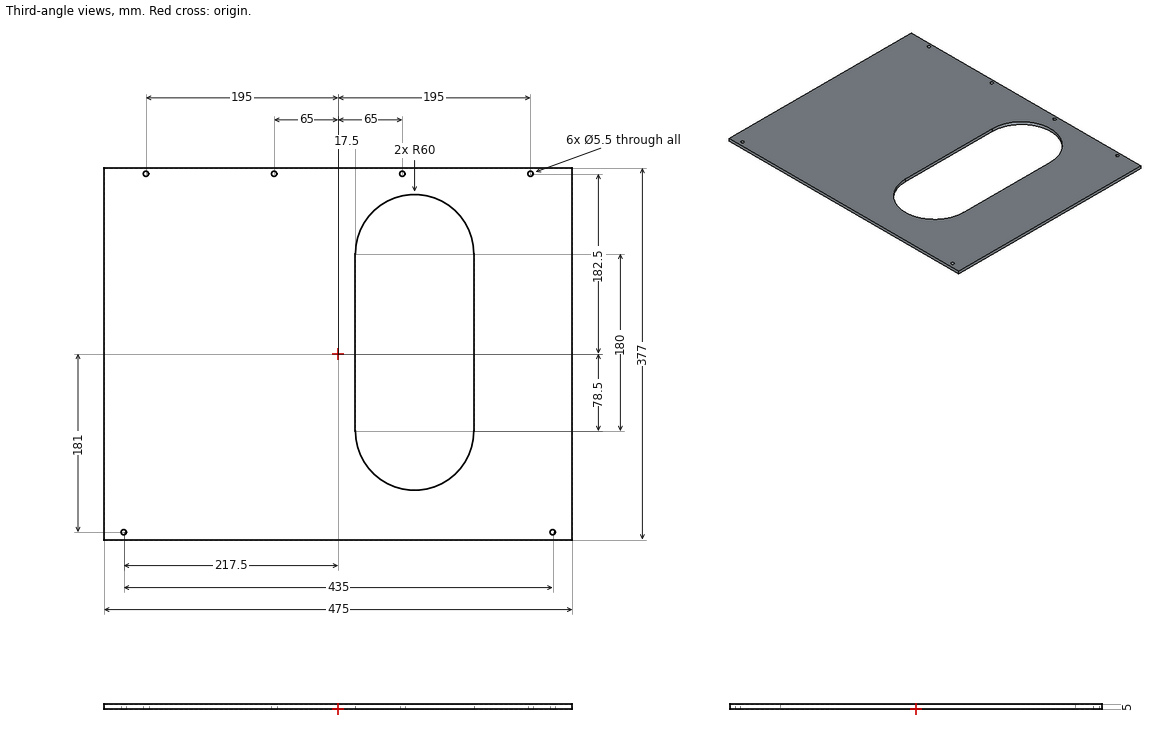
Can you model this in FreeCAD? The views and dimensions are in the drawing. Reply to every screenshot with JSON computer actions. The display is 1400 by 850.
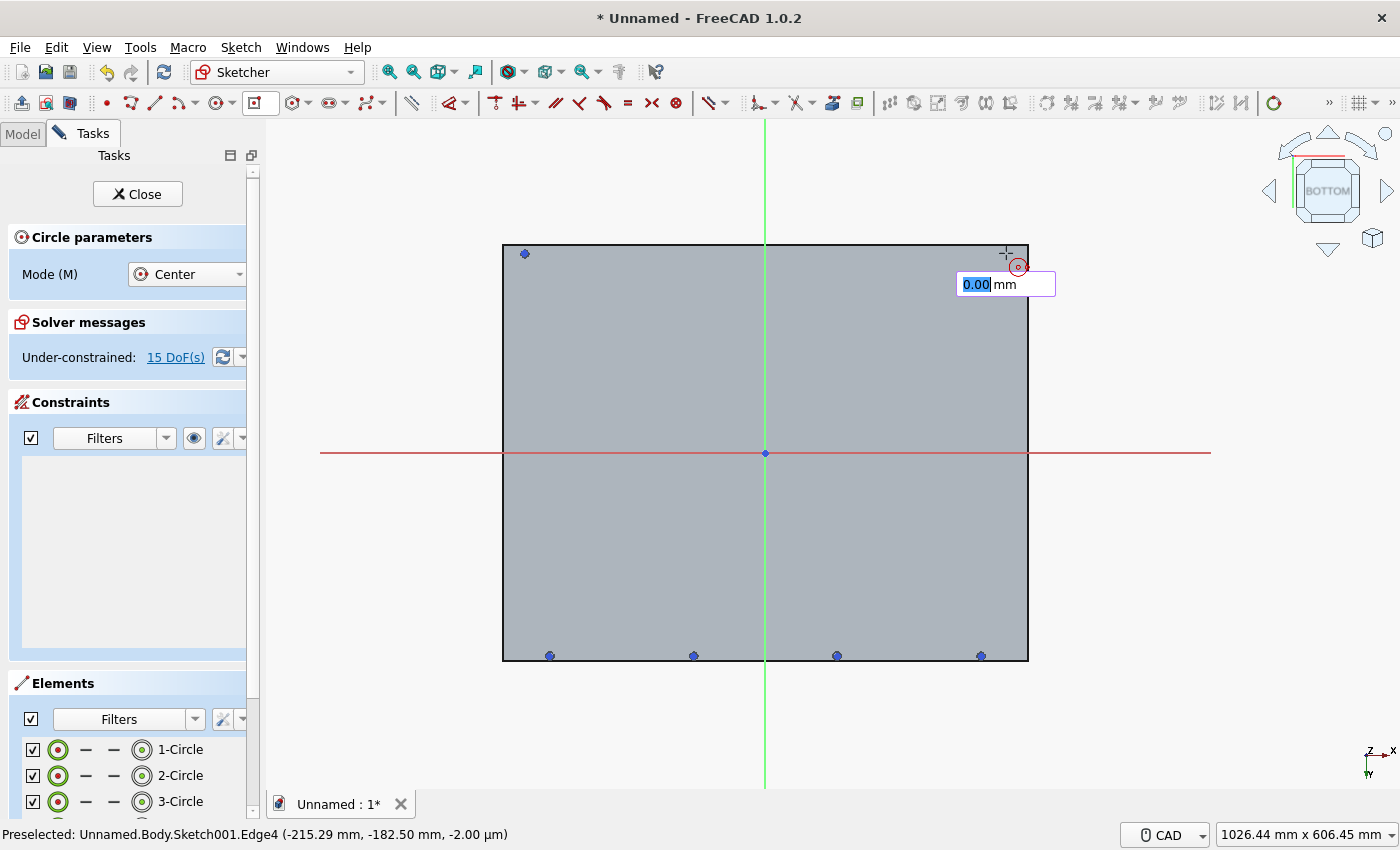
{"action": "scroll", "coordinate": [1008, 251], "scroll_direction": "up", "scroll_amount": 9}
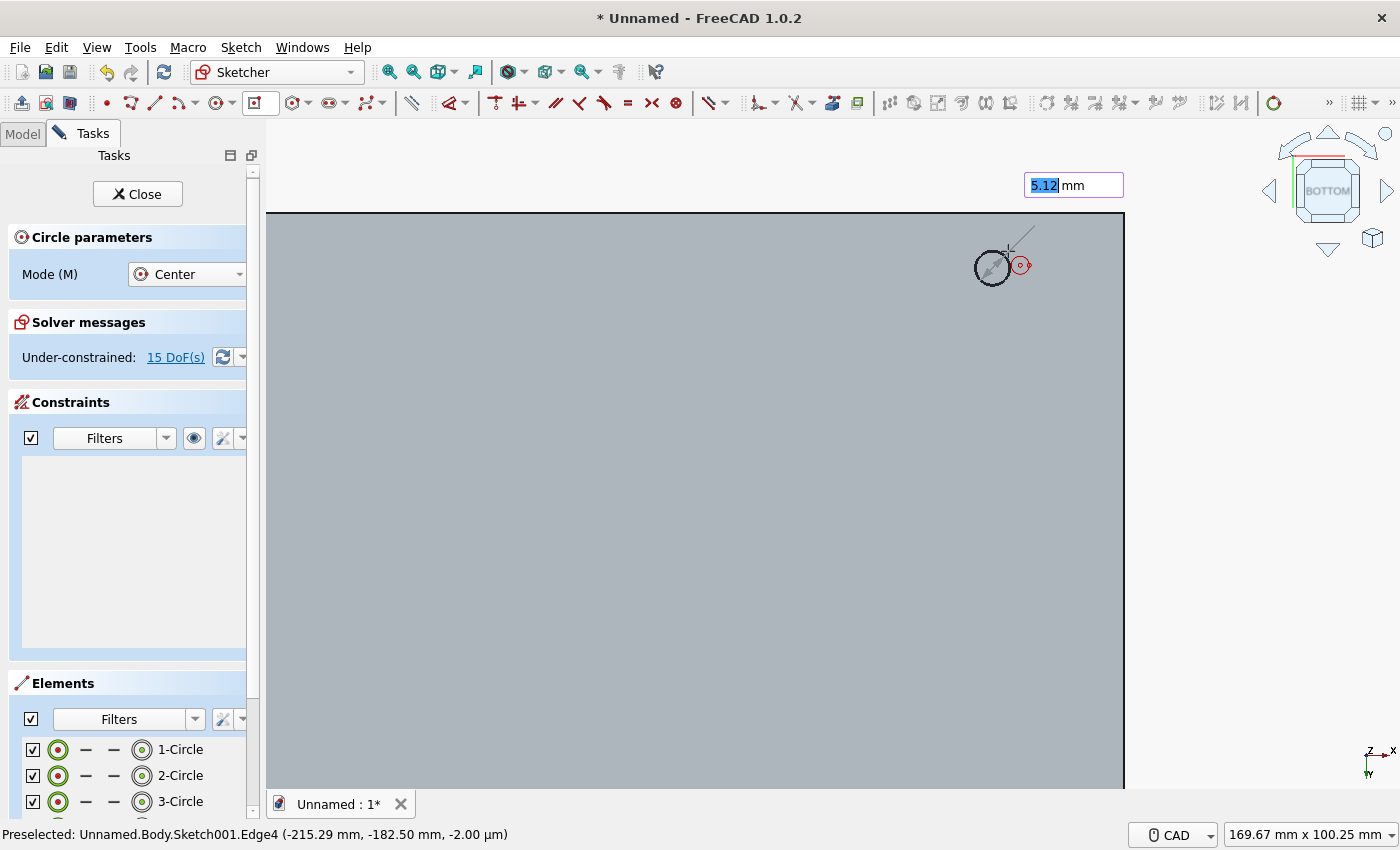
{"action": "left_click", "coordinate": [1004, 250]}
{"action": "key", "text": "Escape"}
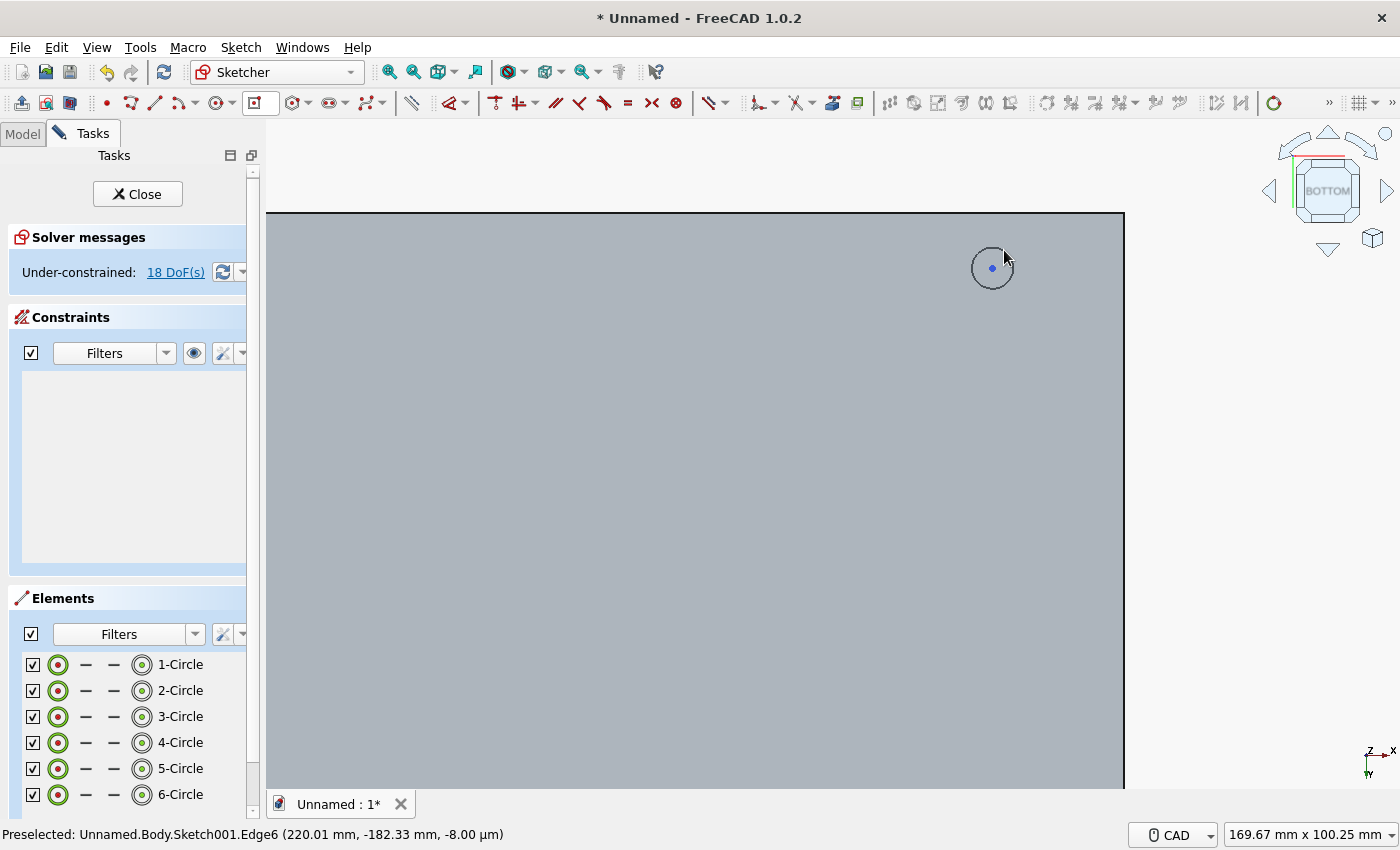
{"action": "scroll", "coordinate": [1008, 251], "scroll_direction": "down", "scroll_amount": 9}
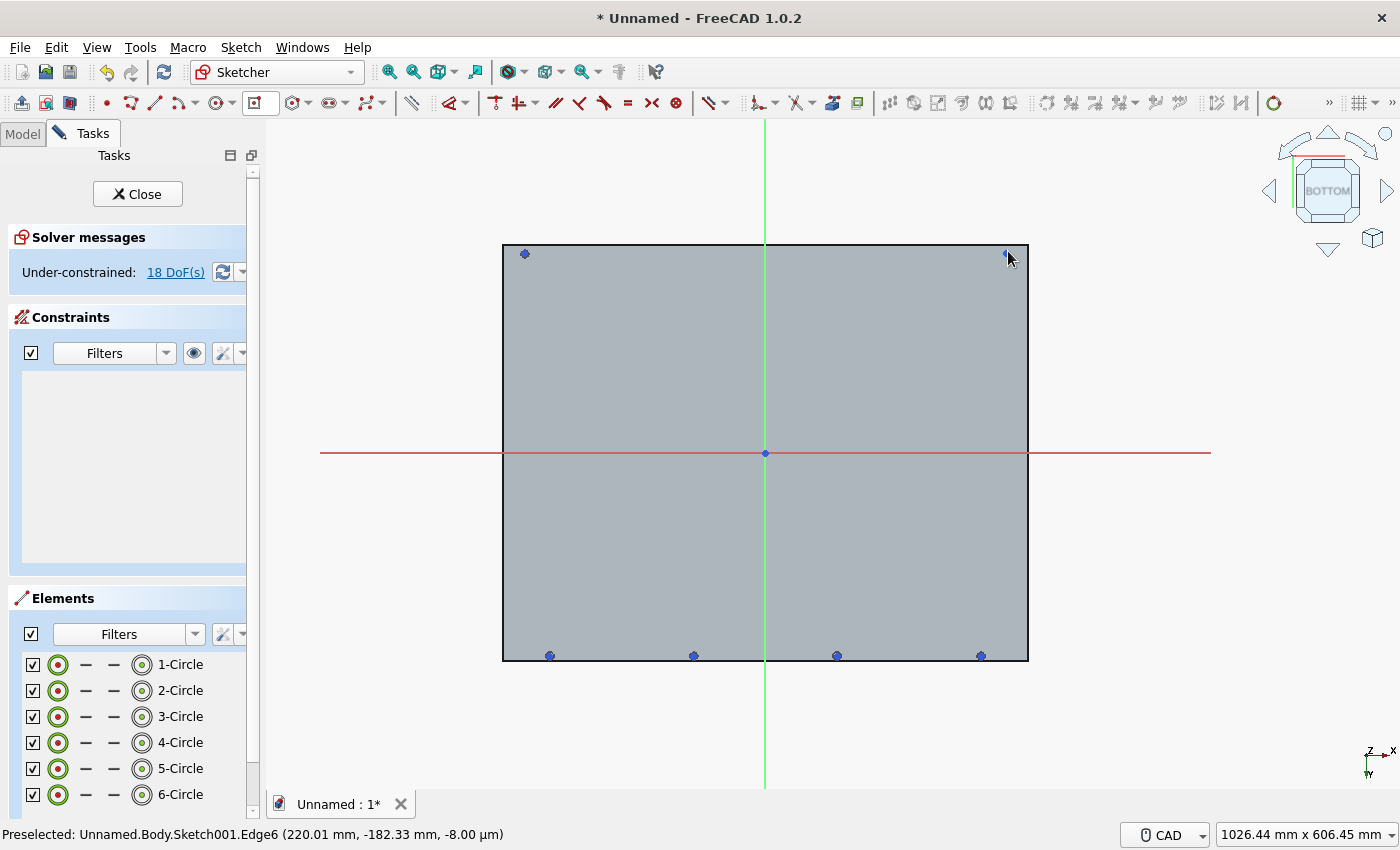
{"action": "scroll", "coordinate": [984, 653], "scroll_direction": "up", "scroll_amount": 7}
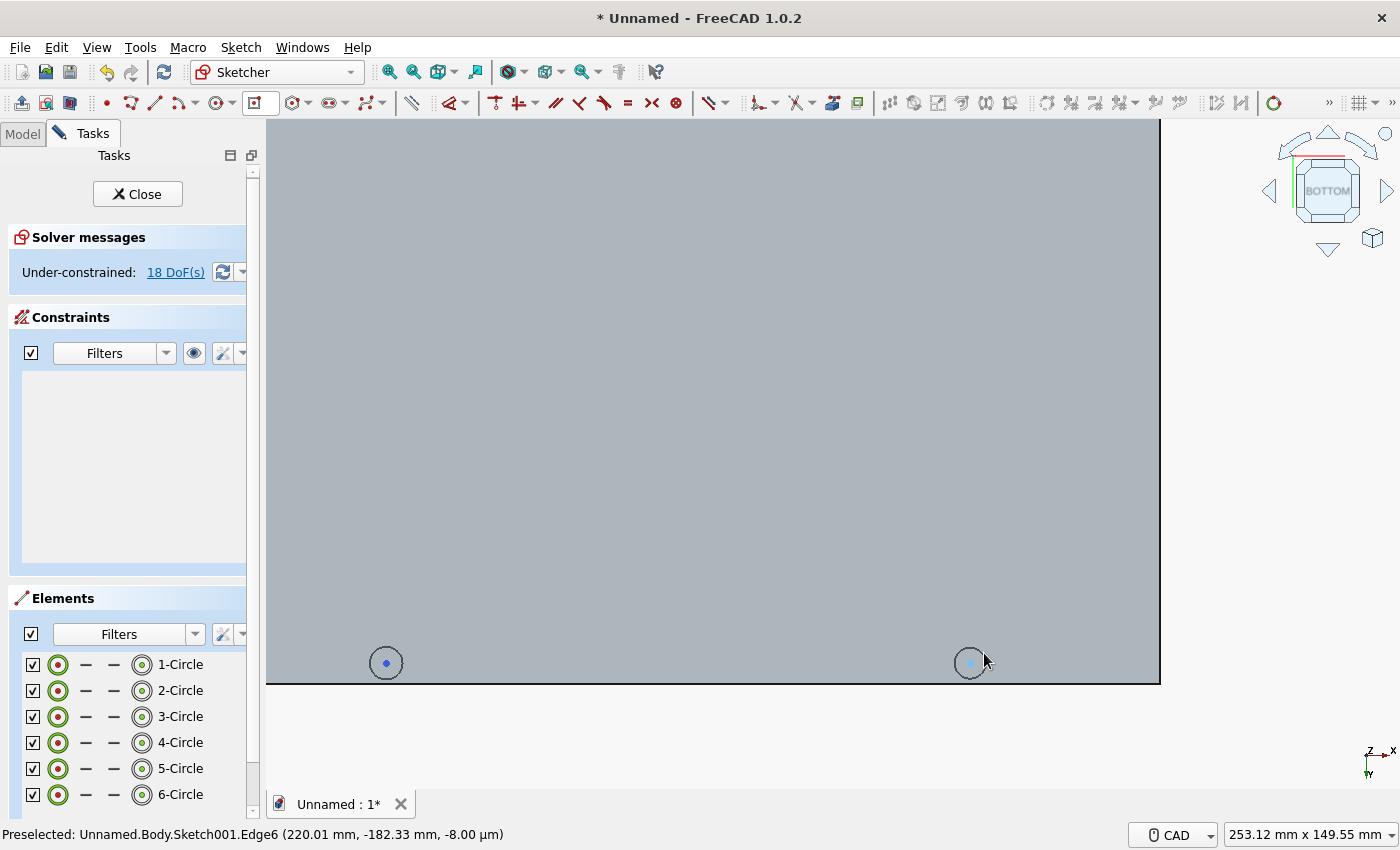
{"action": "left_click", "coordinate": [981, 652]}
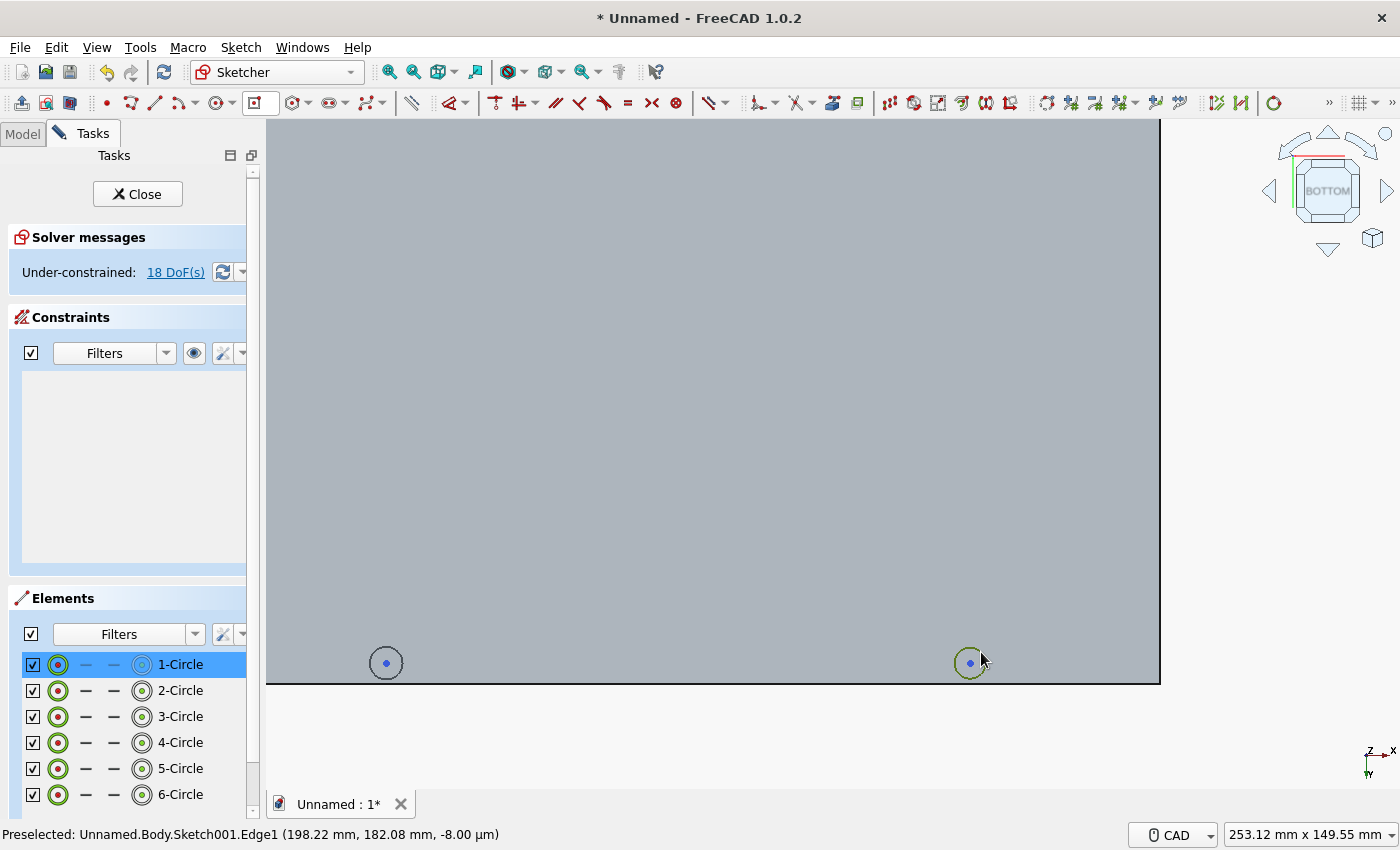
{"action": "left_click", "coordinate": [398, 652]}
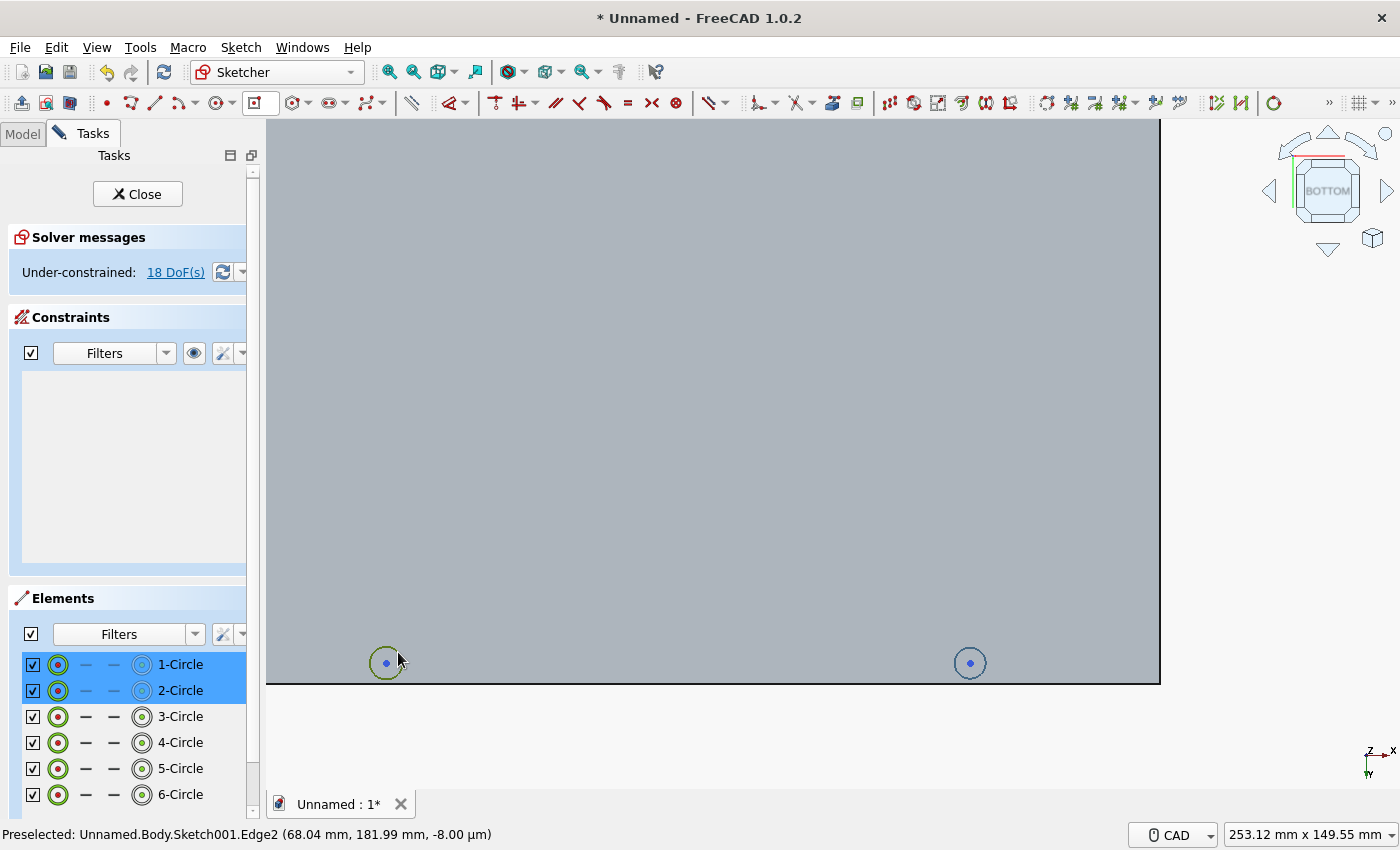
{"action": "scroll", "coordinate": [983, 654], "scroll_direction": "down", "scroll_amount": 7}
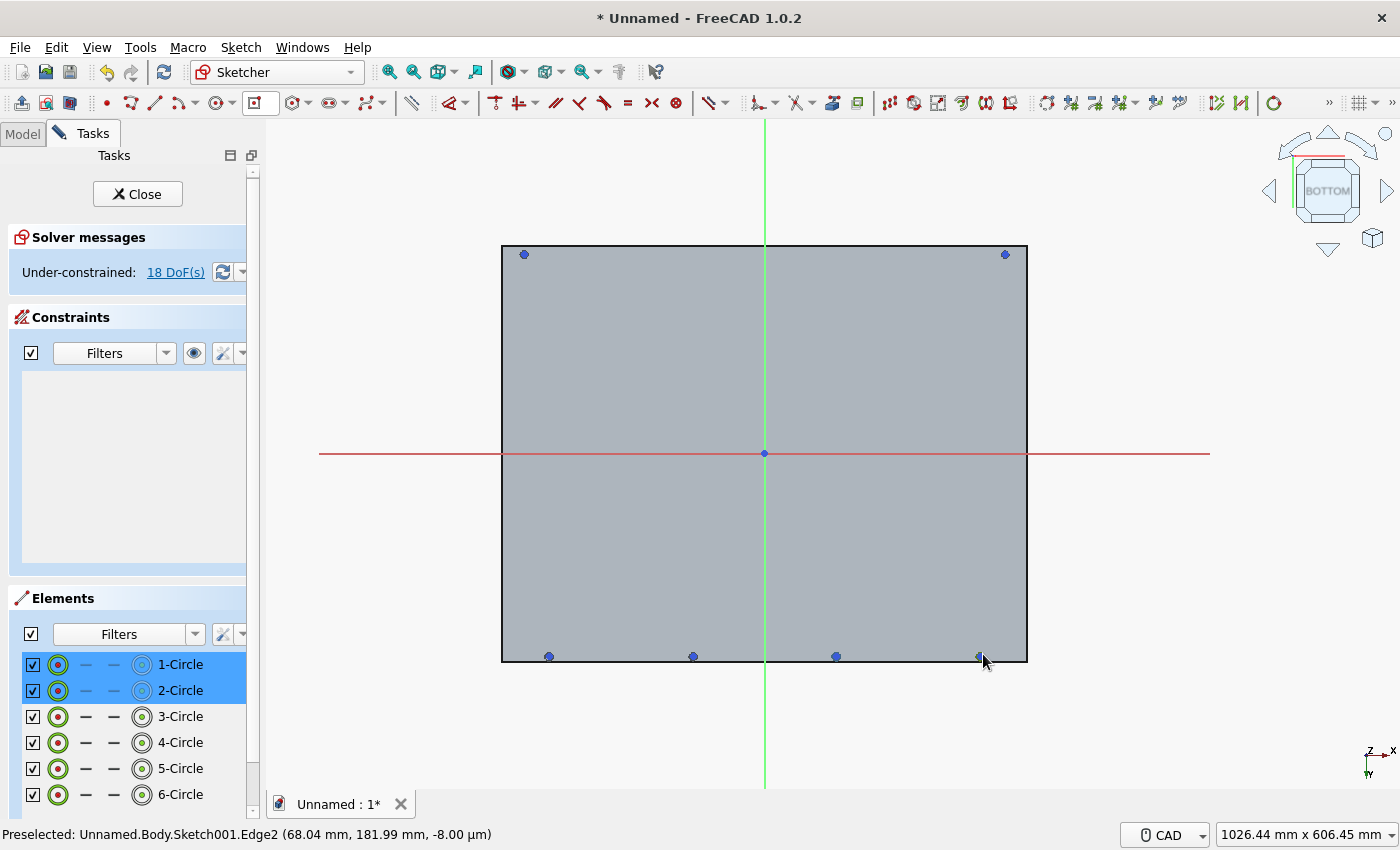
{"action": "scroll", "coordinate": [696, 654], "scroll_direction": "up", "scroll_amount": 7}